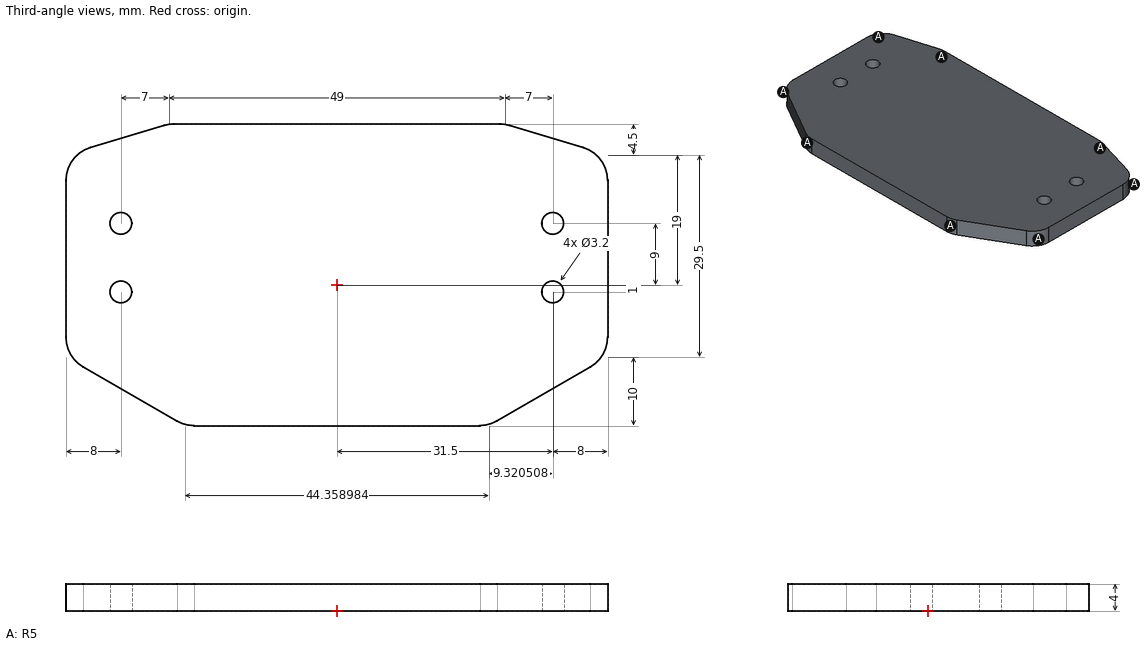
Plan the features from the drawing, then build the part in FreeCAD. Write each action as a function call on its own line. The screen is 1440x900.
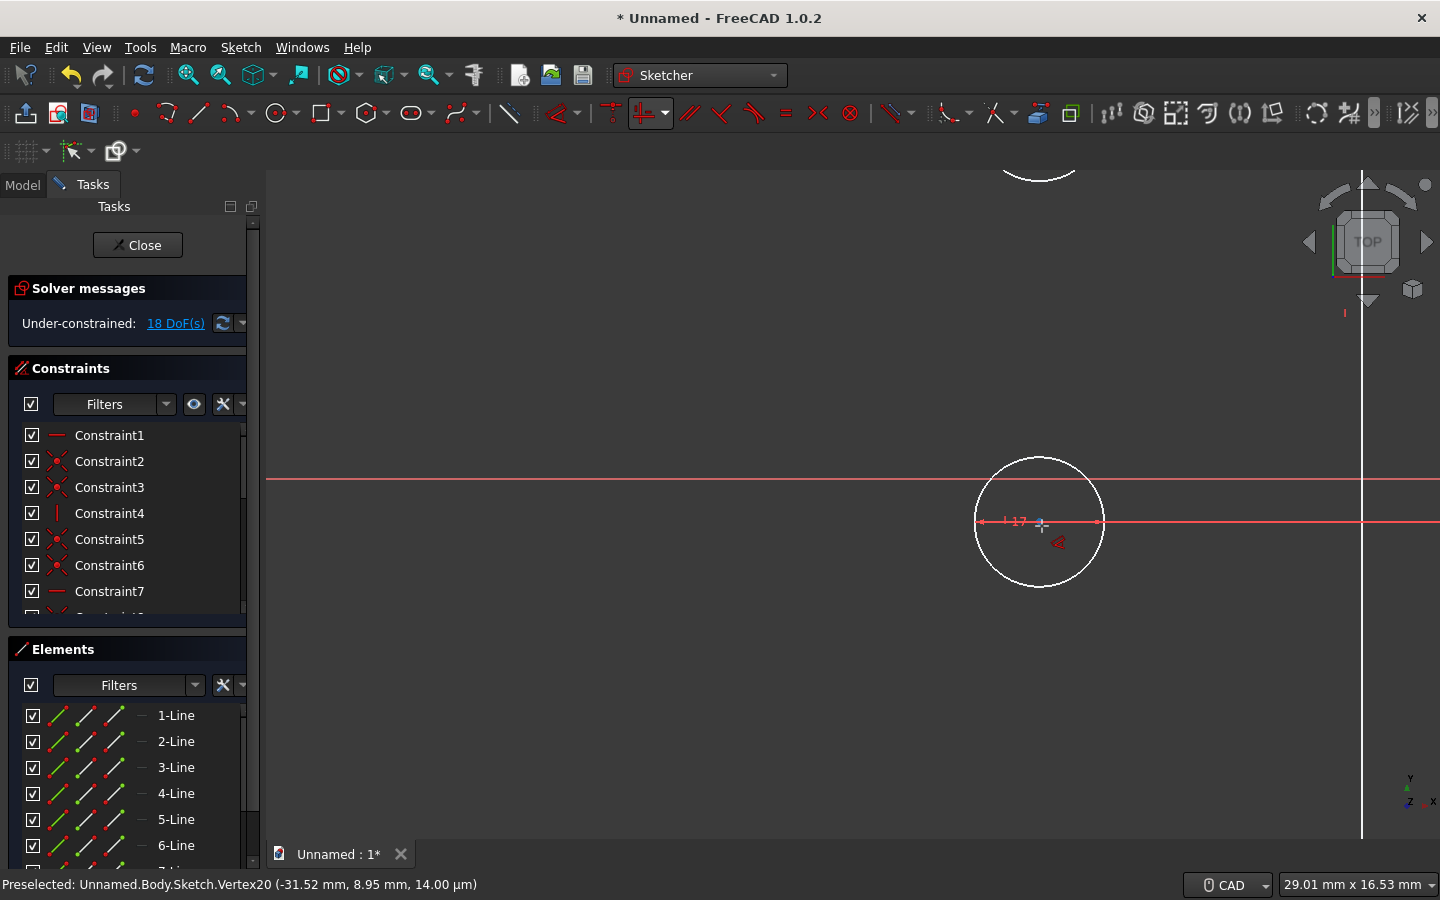
click(1039, 522)
click(1073, 500)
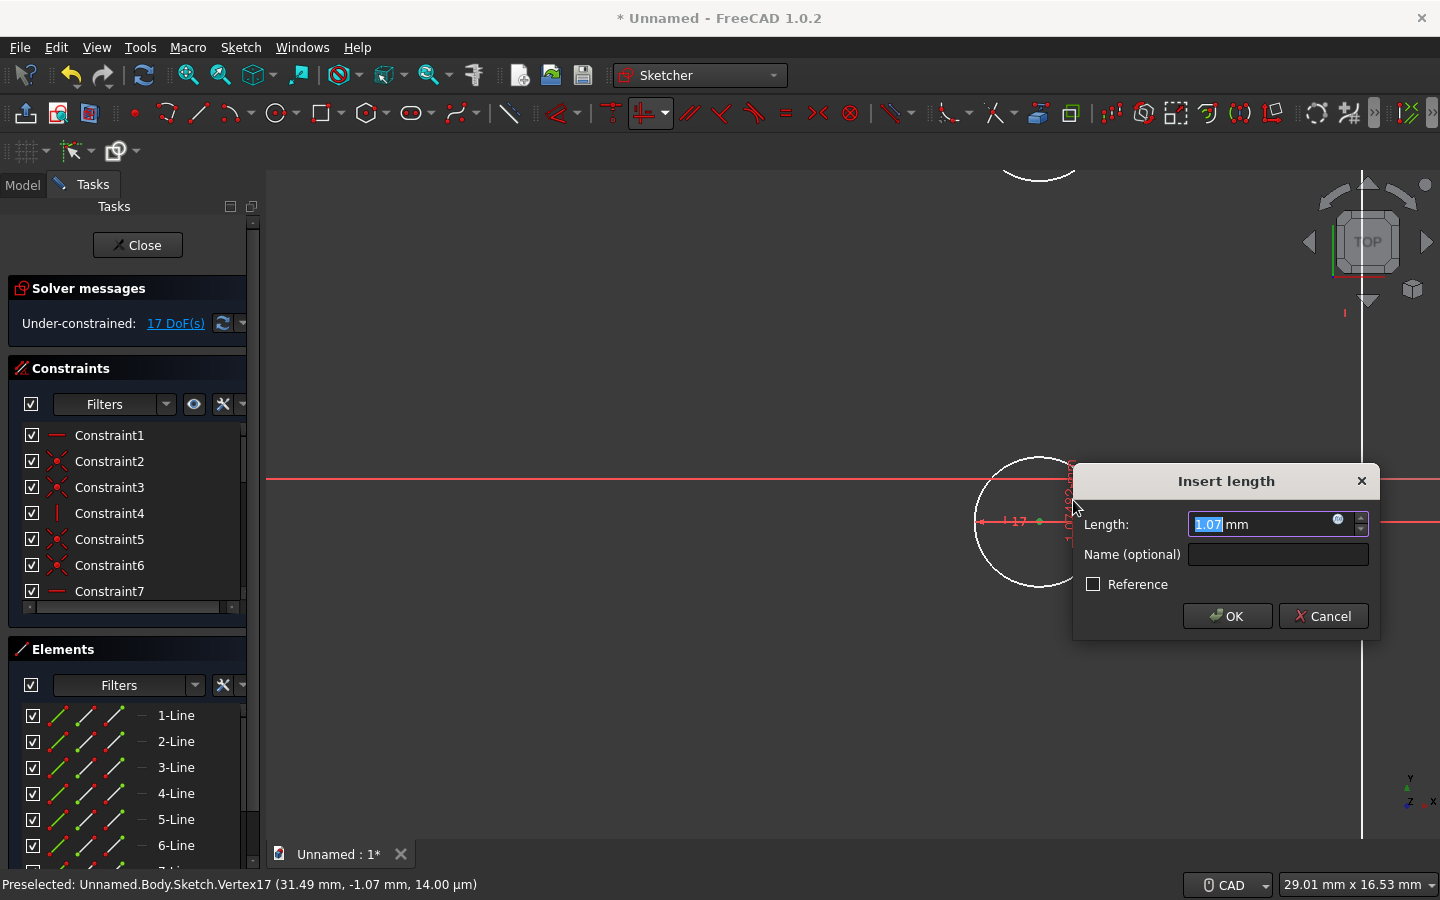
text(1)
key(Return)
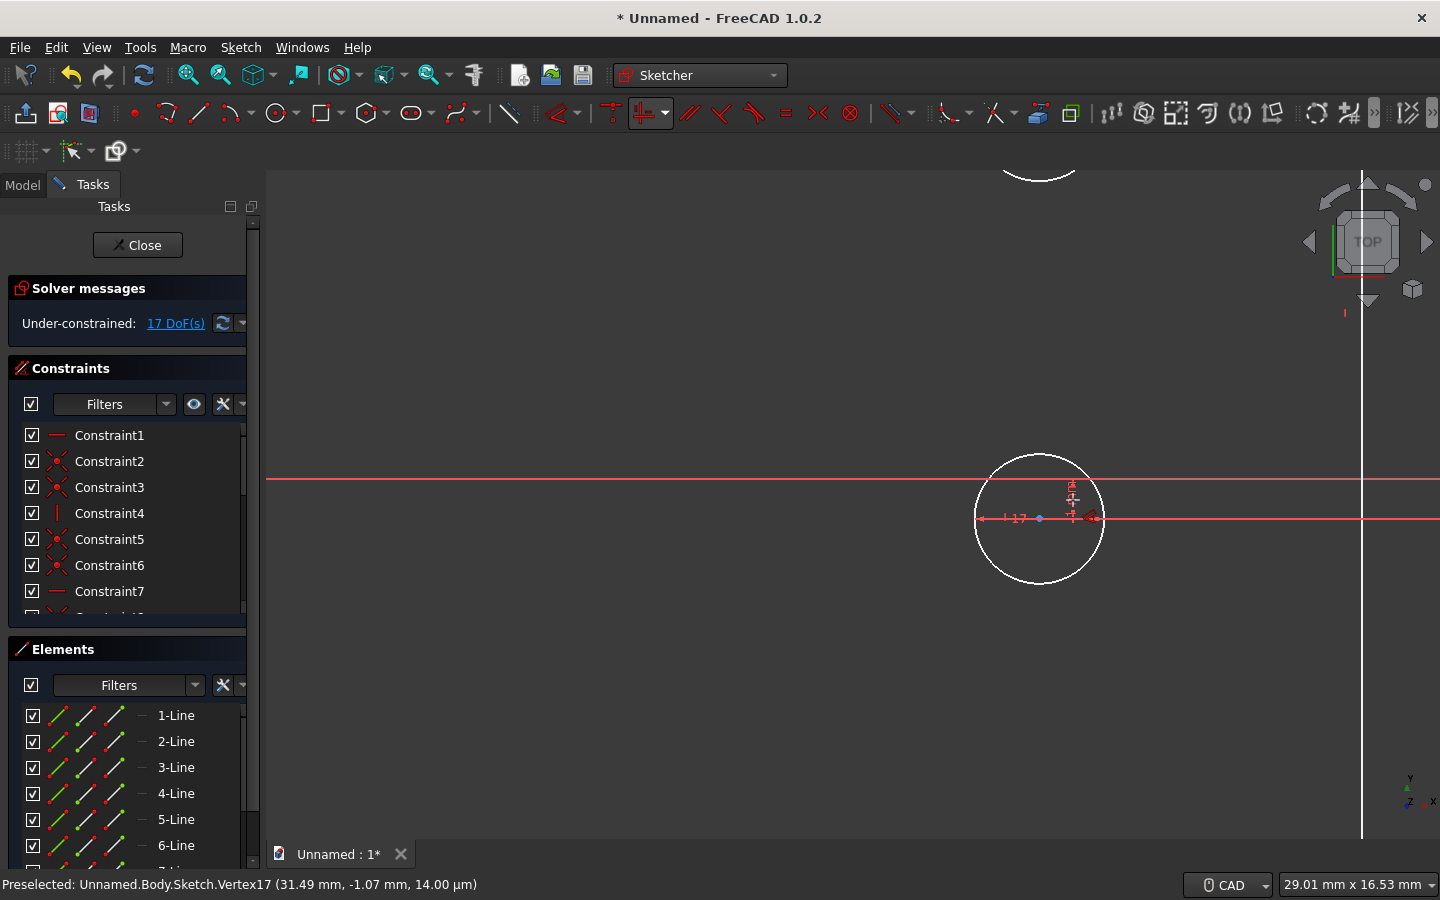
scroll(1042, 526, down, 8)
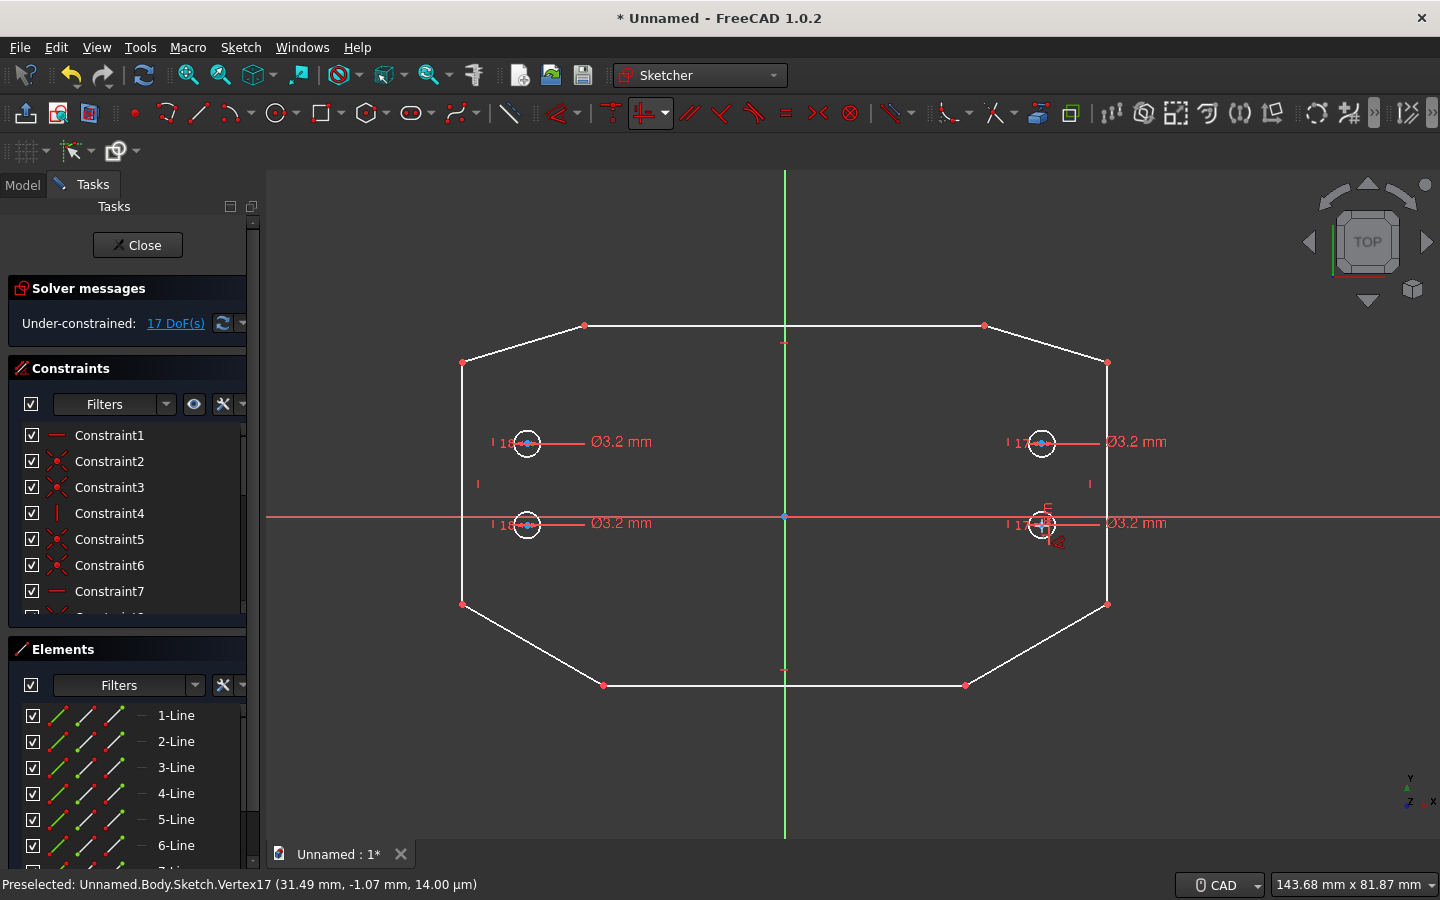
scroll(527, 525, up, 8)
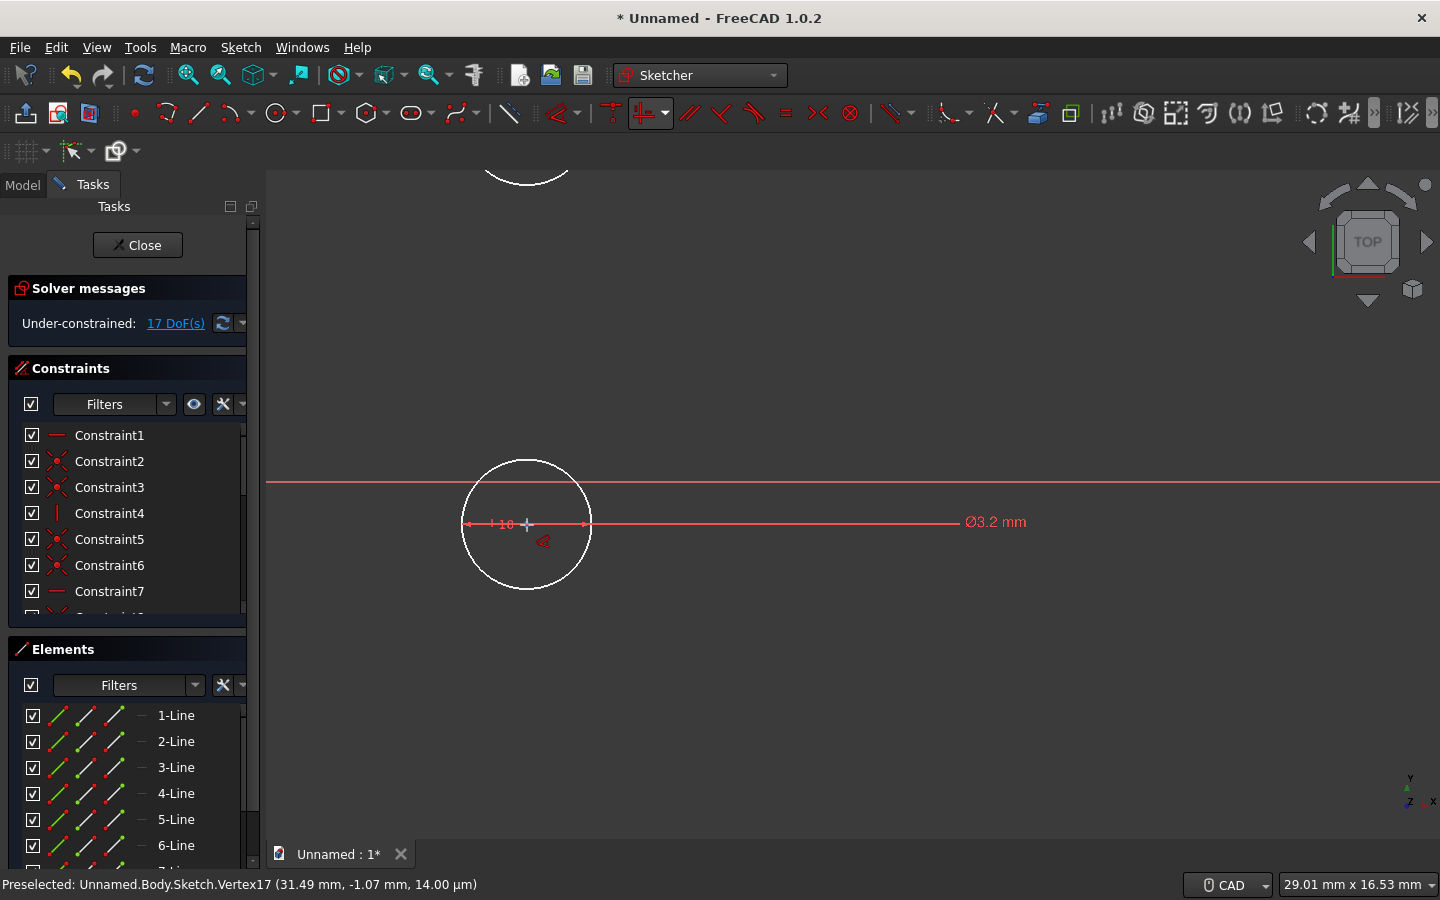
click(527, 524)
click(493, 503)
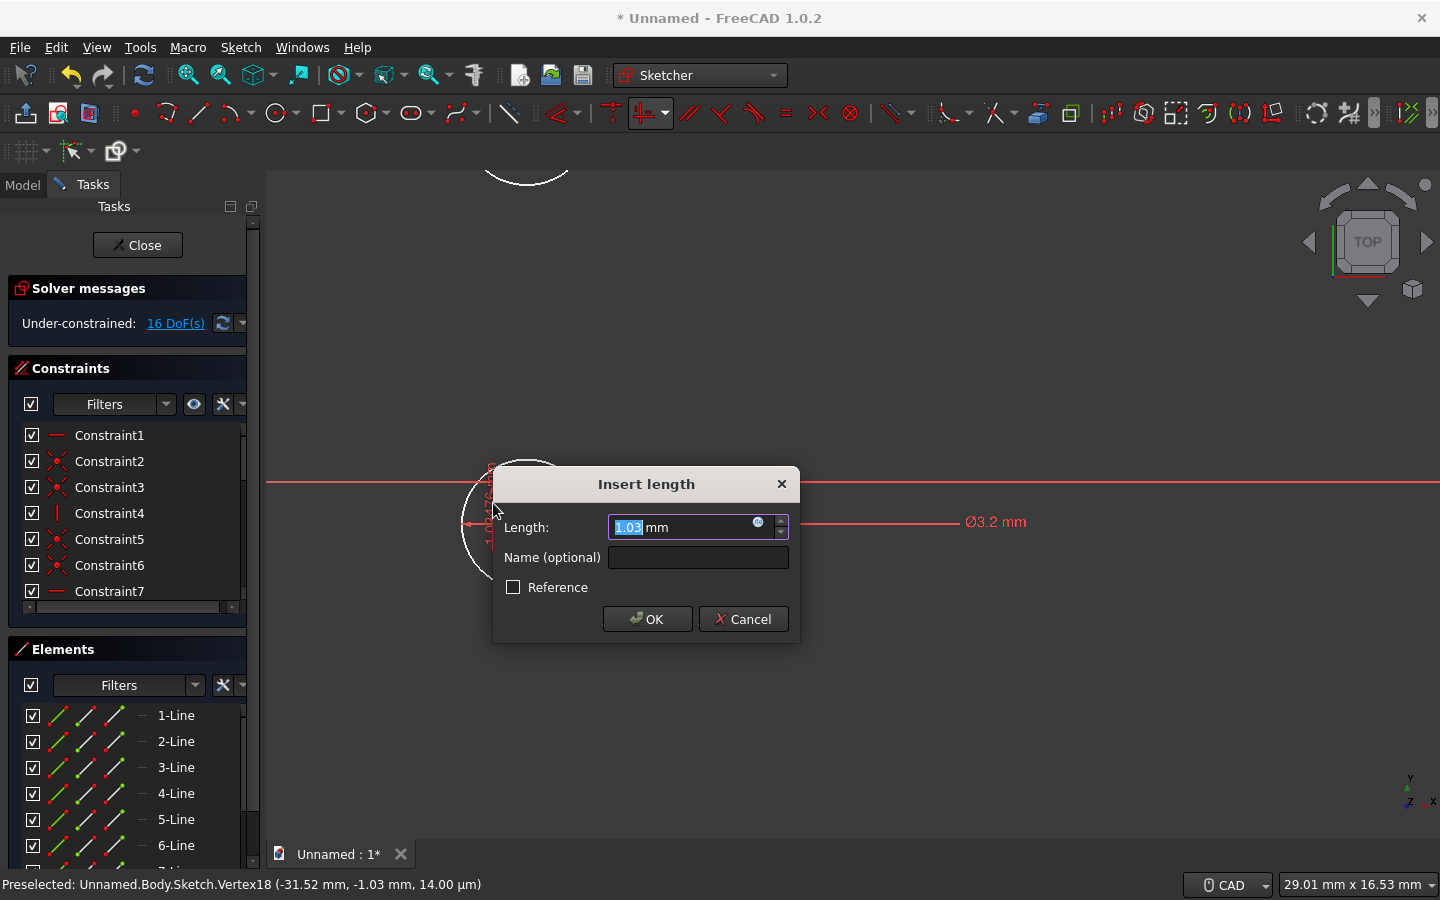
text(1)
key(Return)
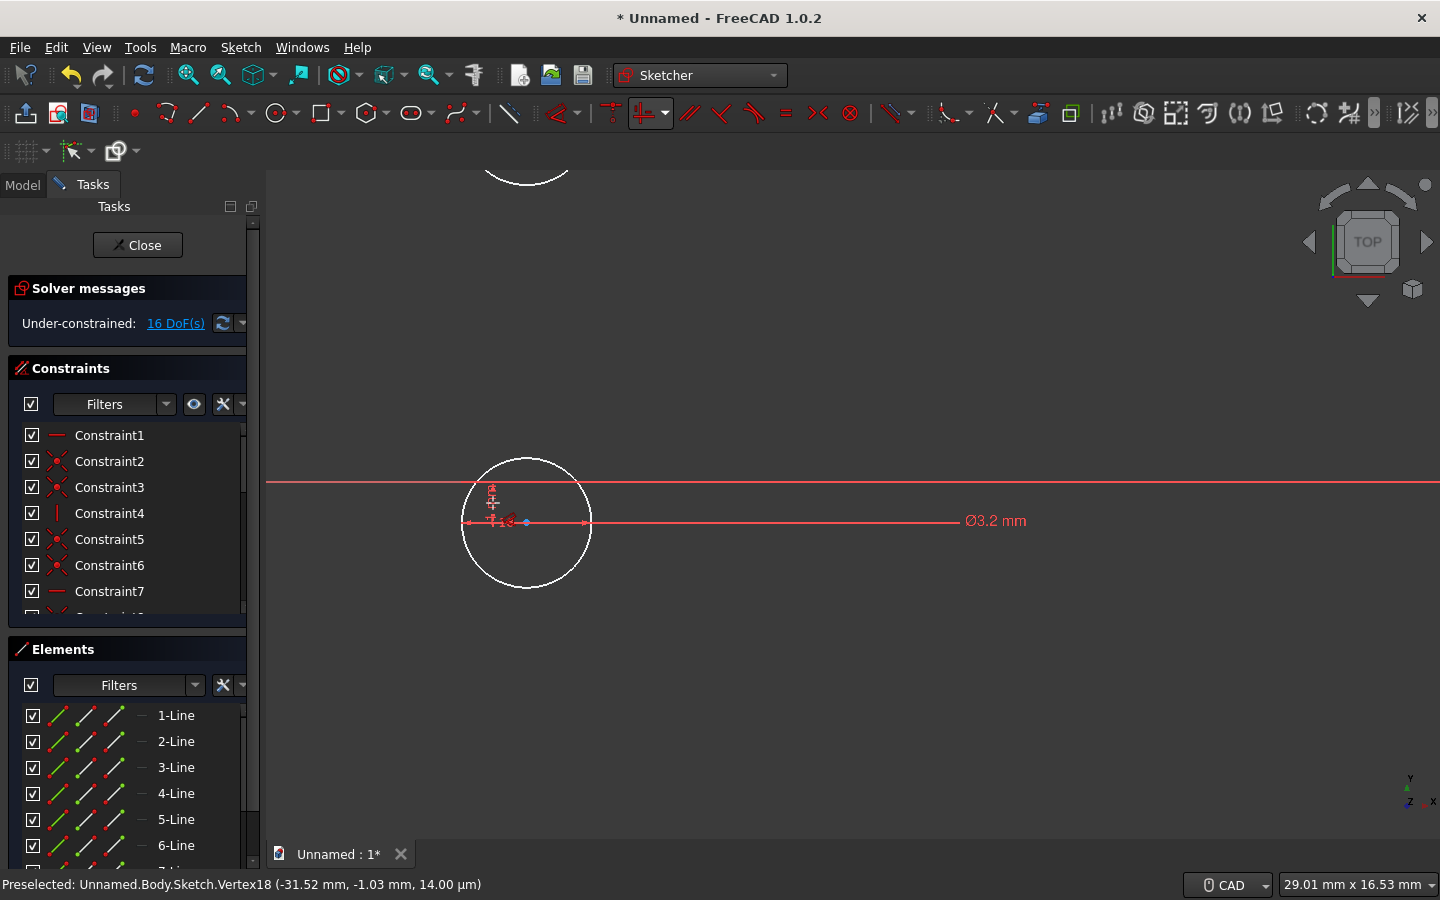
scroll(527, 525, down, 8)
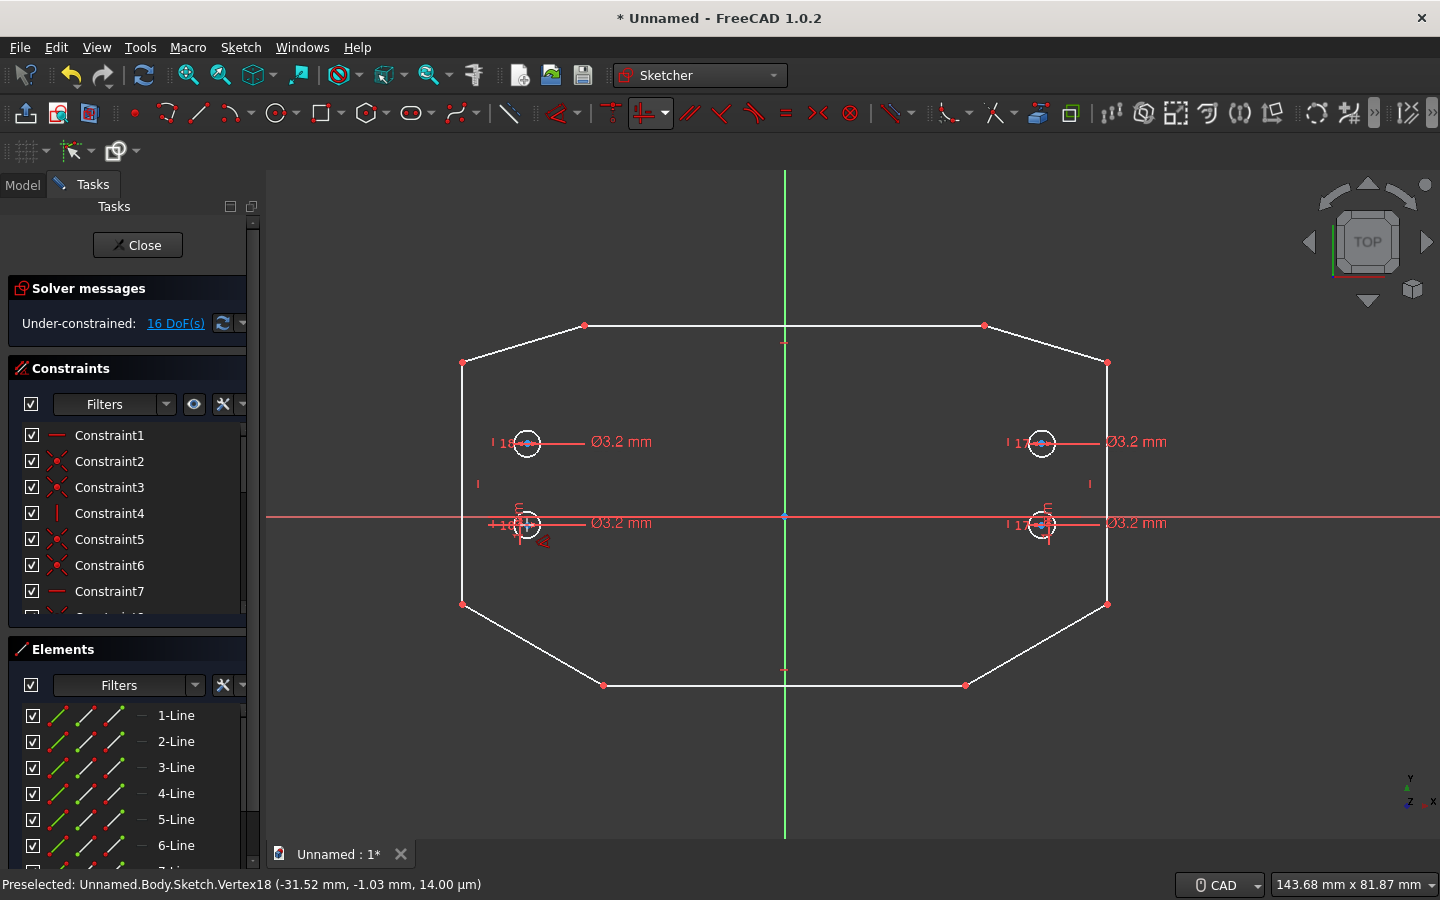
click(1042, 444)
click(1076, 480)